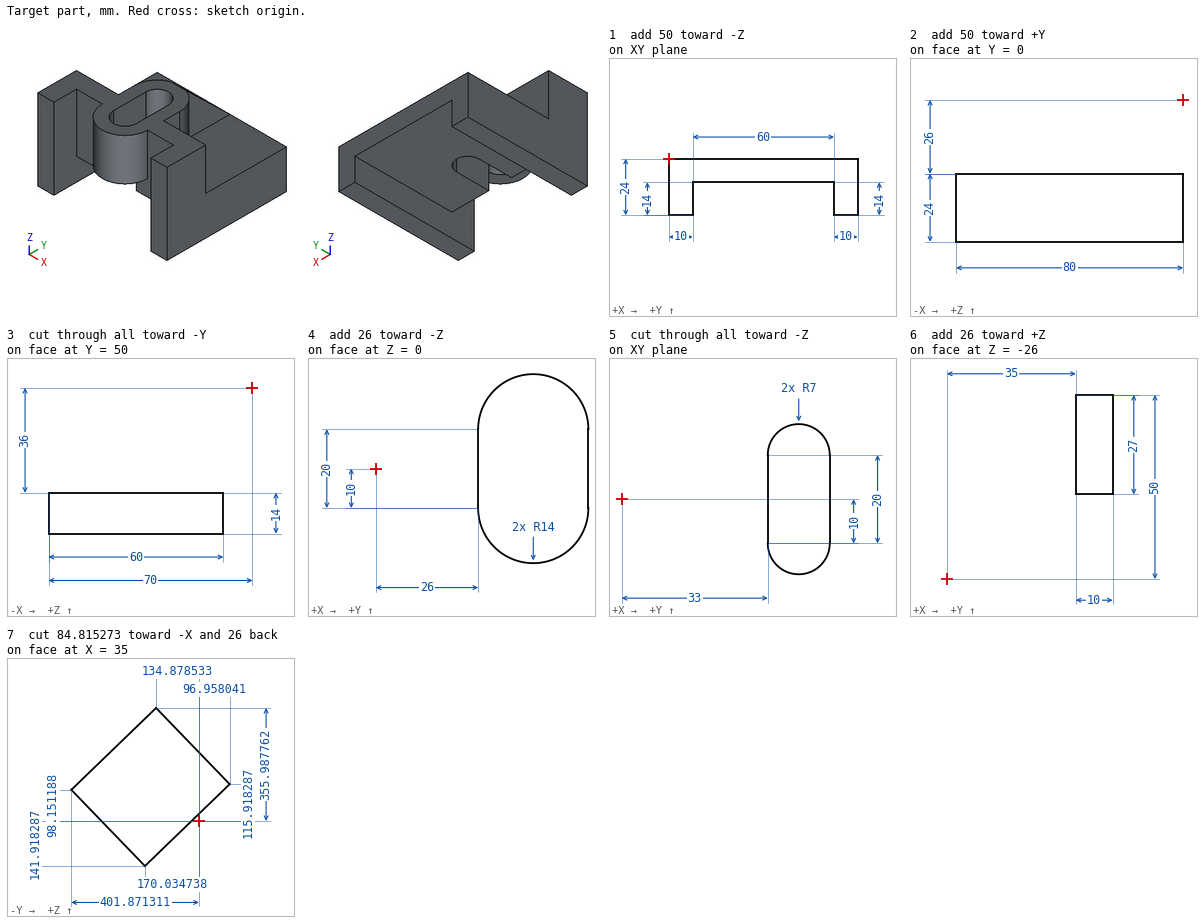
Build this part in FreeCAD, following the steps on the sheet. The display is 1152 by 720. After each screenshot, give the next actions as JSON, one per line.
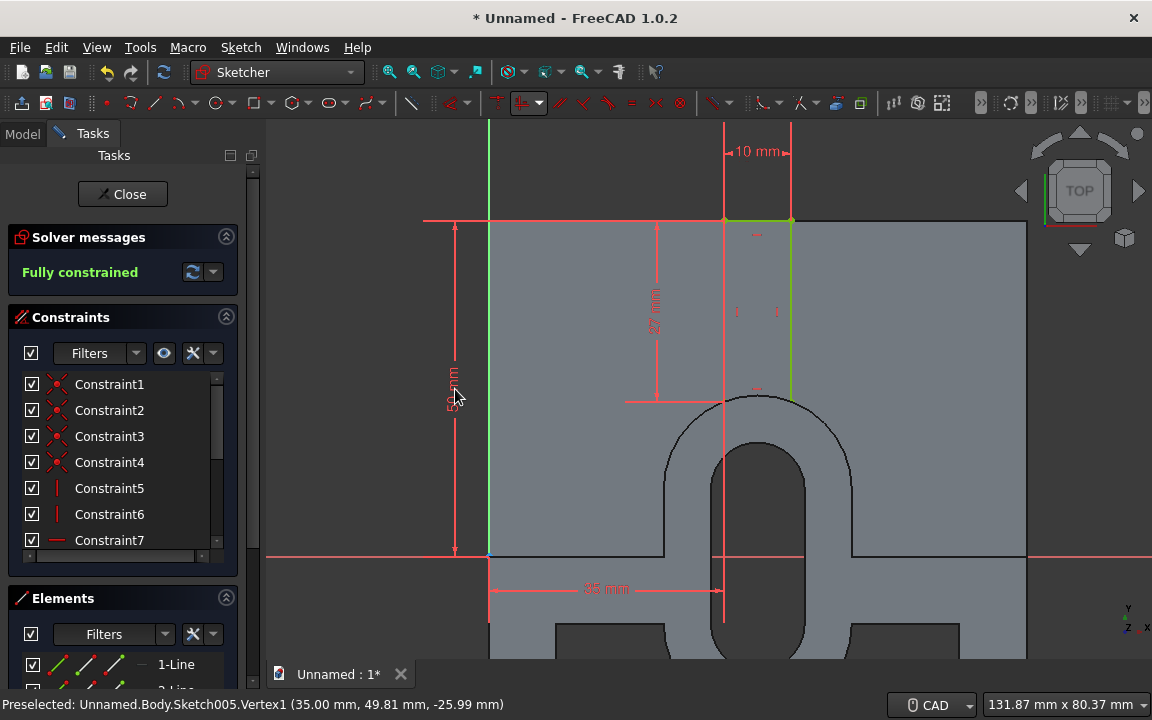
{"action": "left_click", "coordinate": [123, 194]}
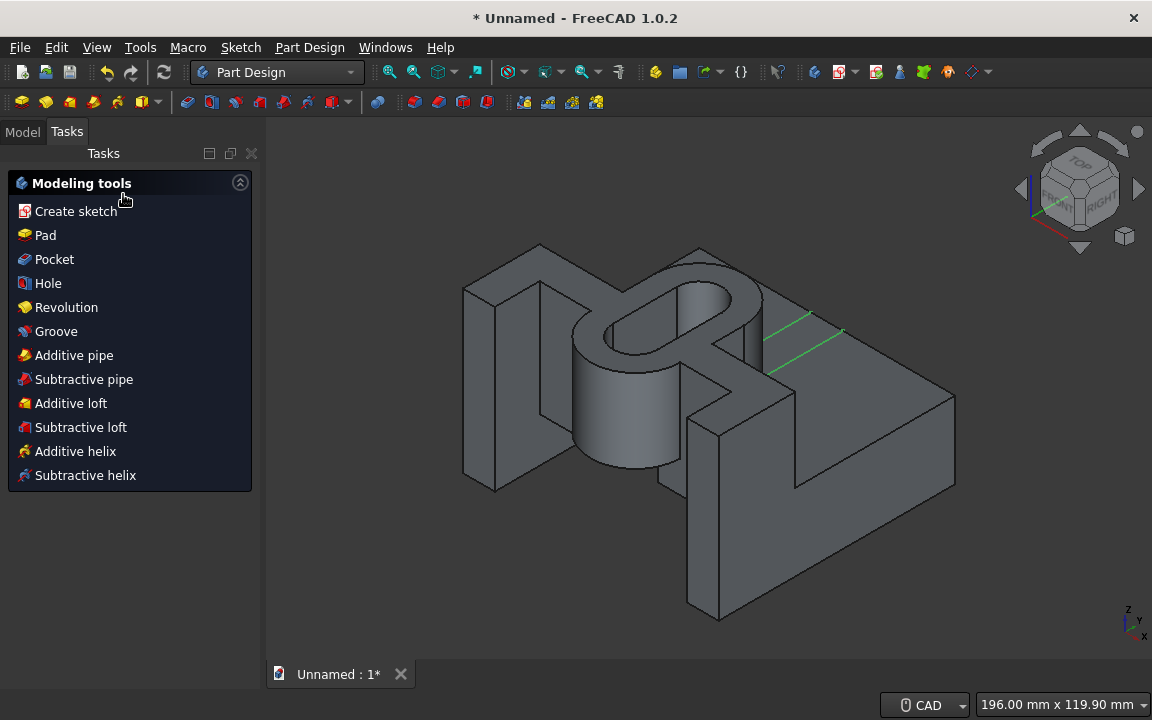
{"action": "left_click", "coordinate": [22, 102]}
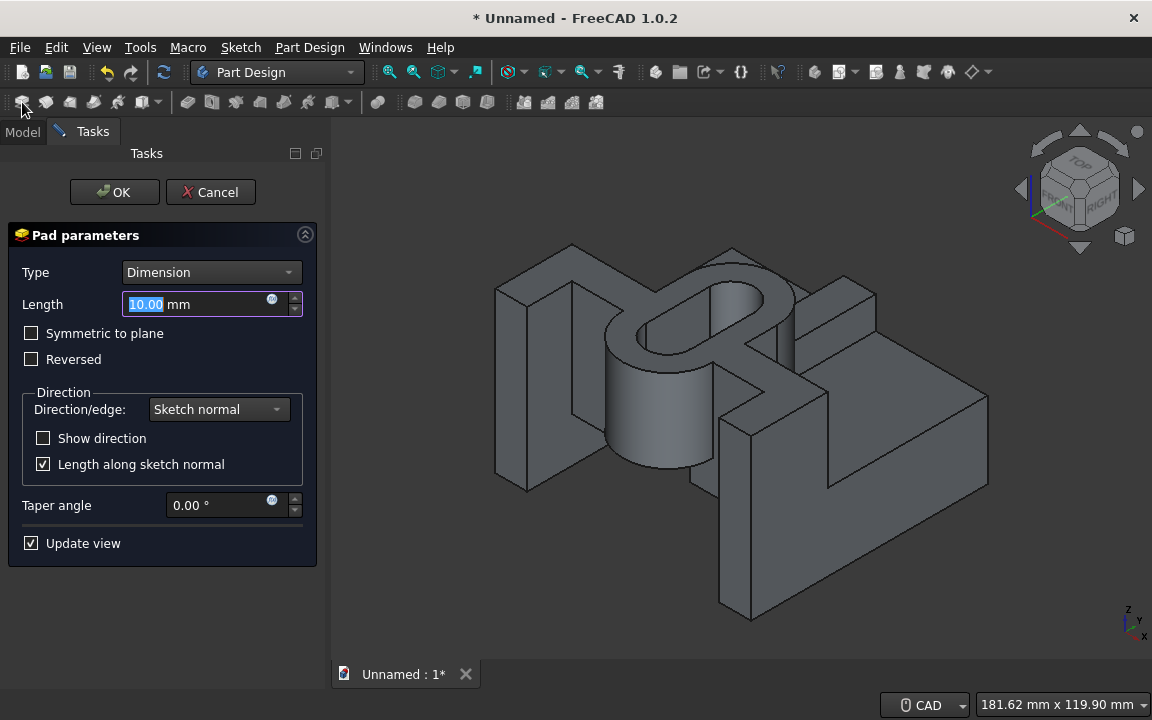
{"action": "type", "text": "26"}
{"action": "key", "text": "Tab"}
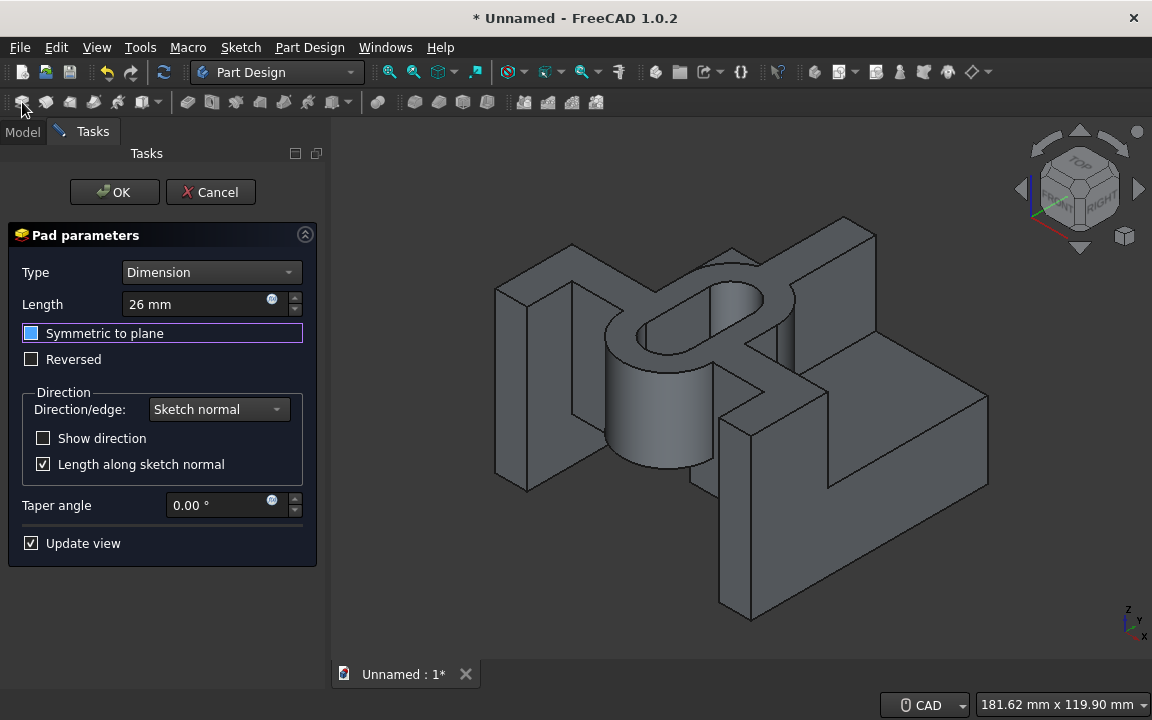
{"action": "left_click", "coordinate": [115, 192]}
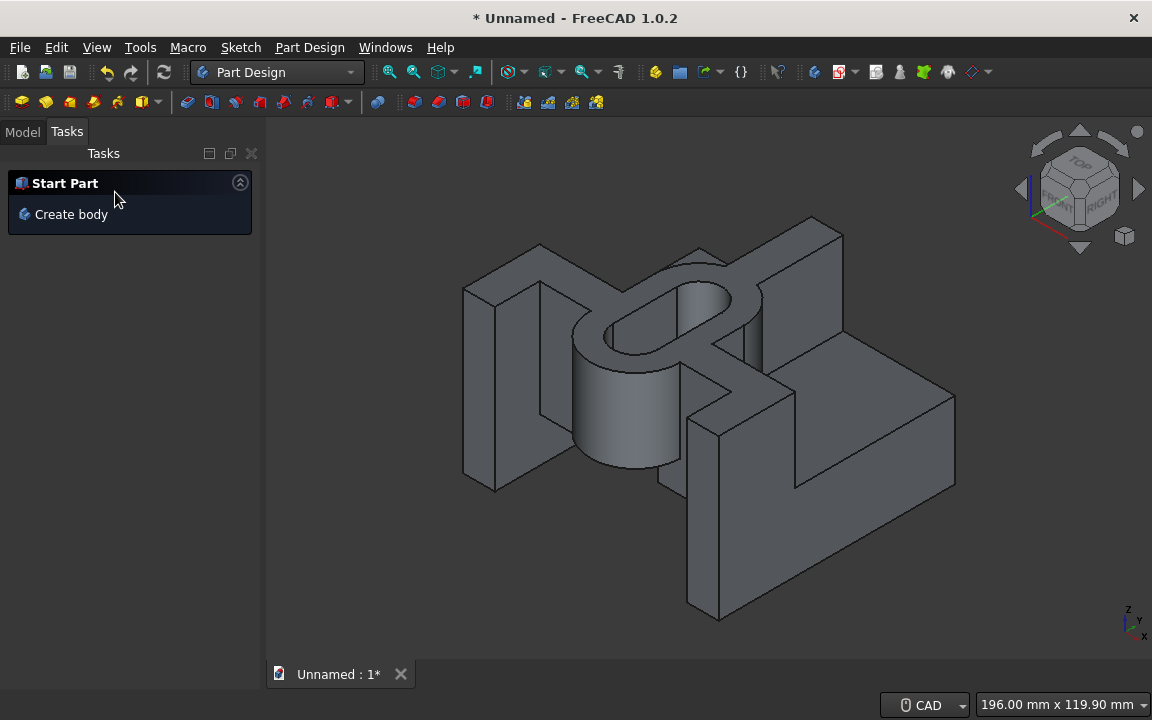
{"action": "key", "text": "6"}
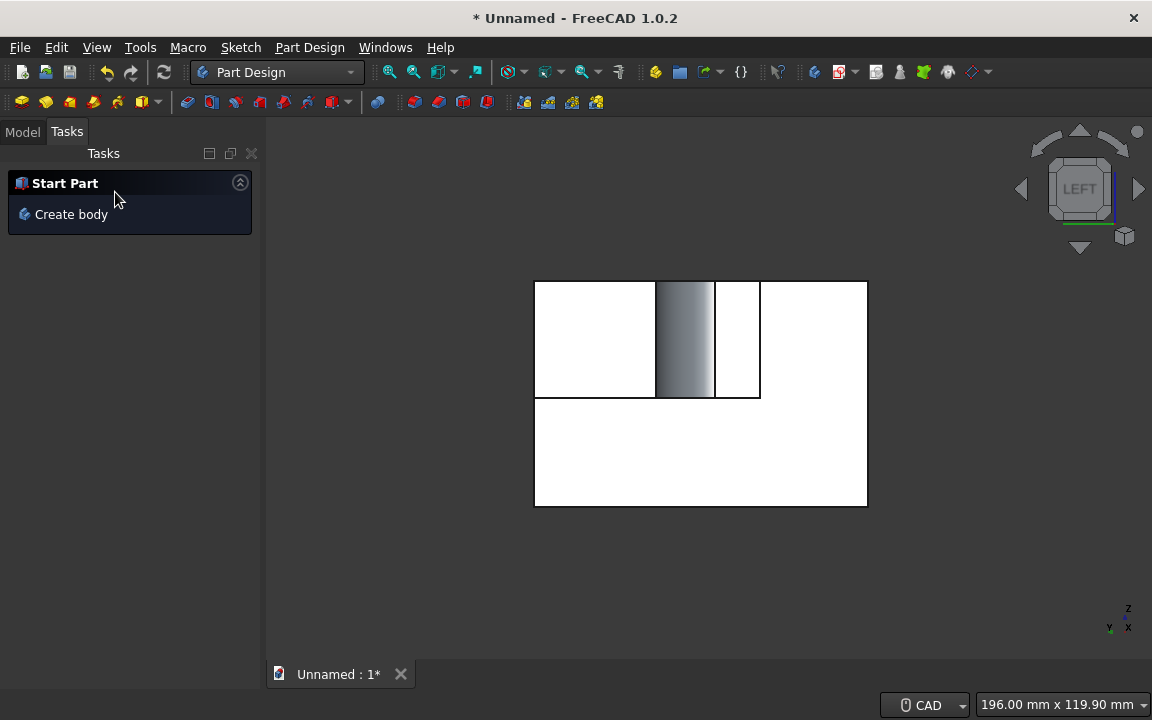
{"action": "key", "text": "v f"}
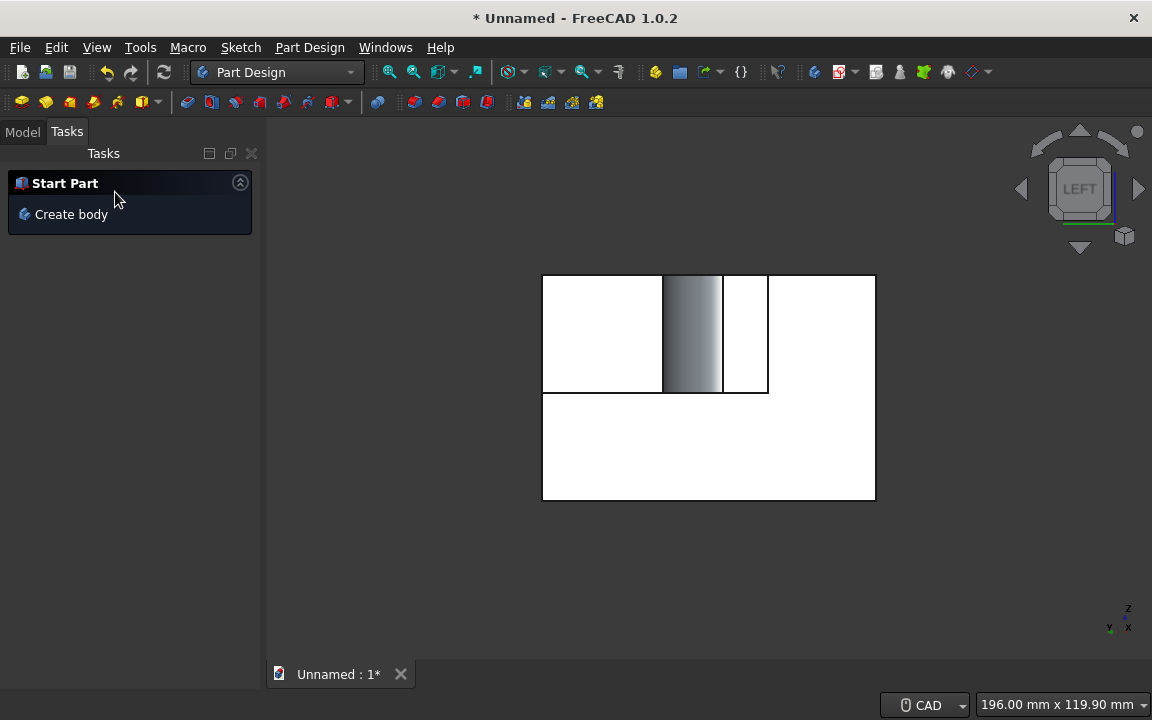
{"action": "left_click", "coordinate": [603, 333]}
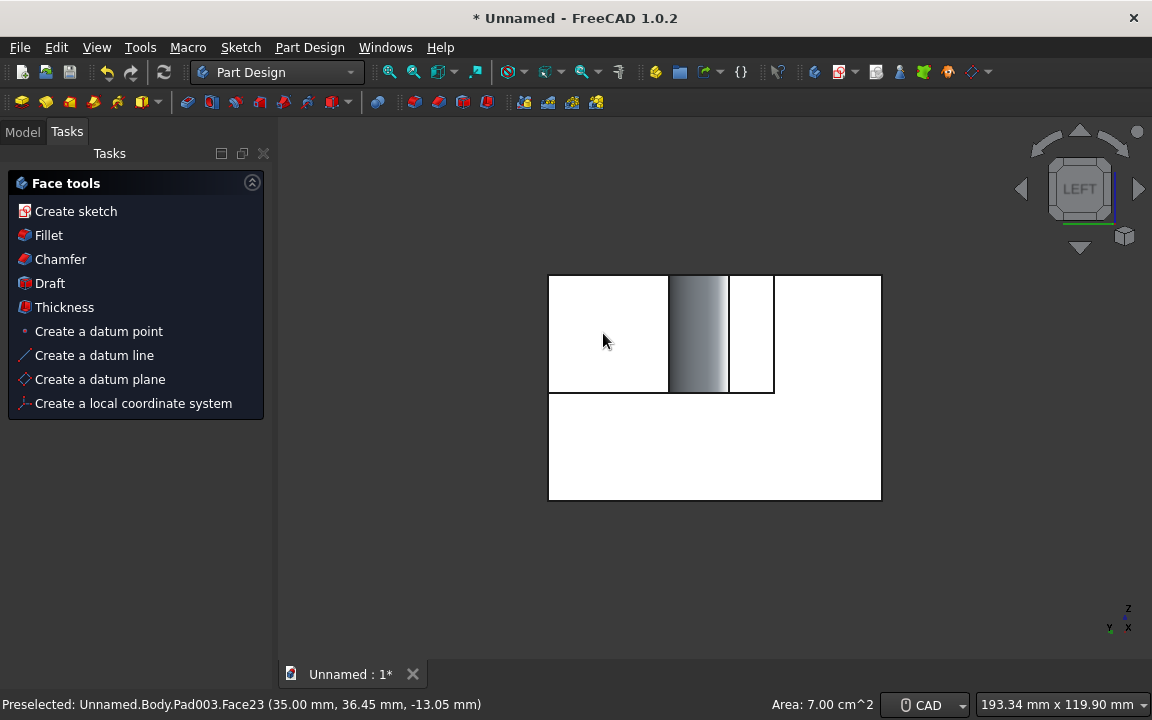
{"action": "left_click", "coordinate": [840, 72]}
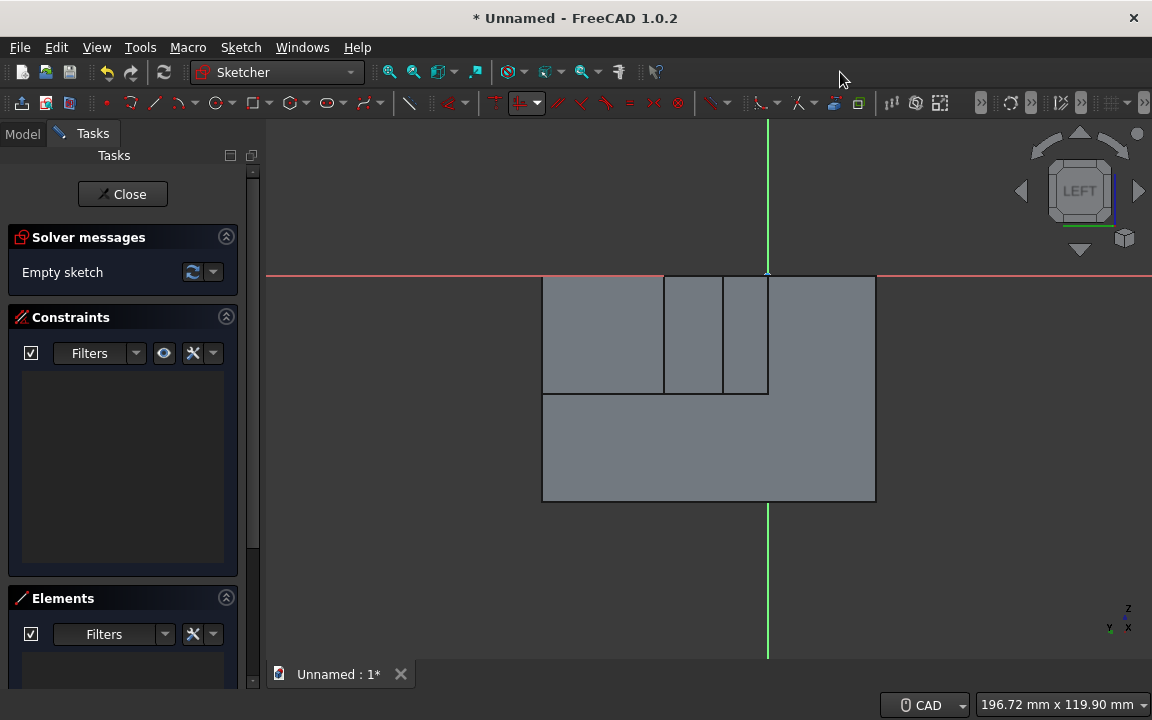
{"action": "scroll", "coordinate": [751, 507], "scroll_direction": "down", "scroll_amount": 9}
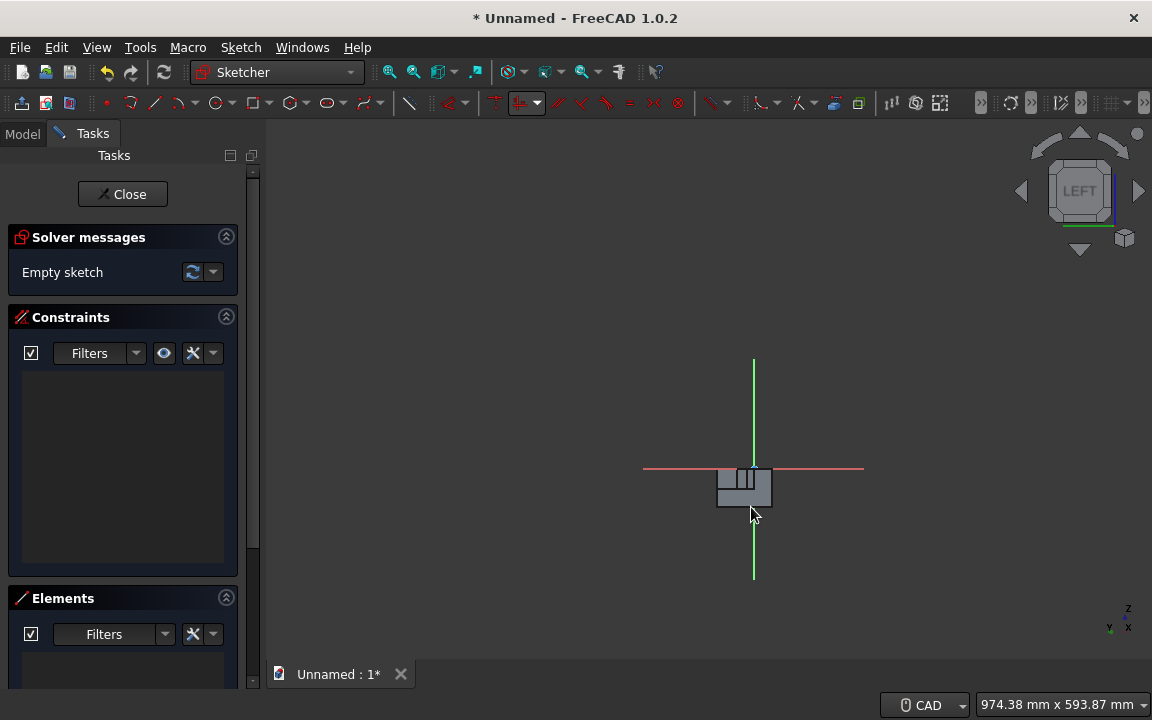
{"action": "left_click", "coordinate": [132, 104]}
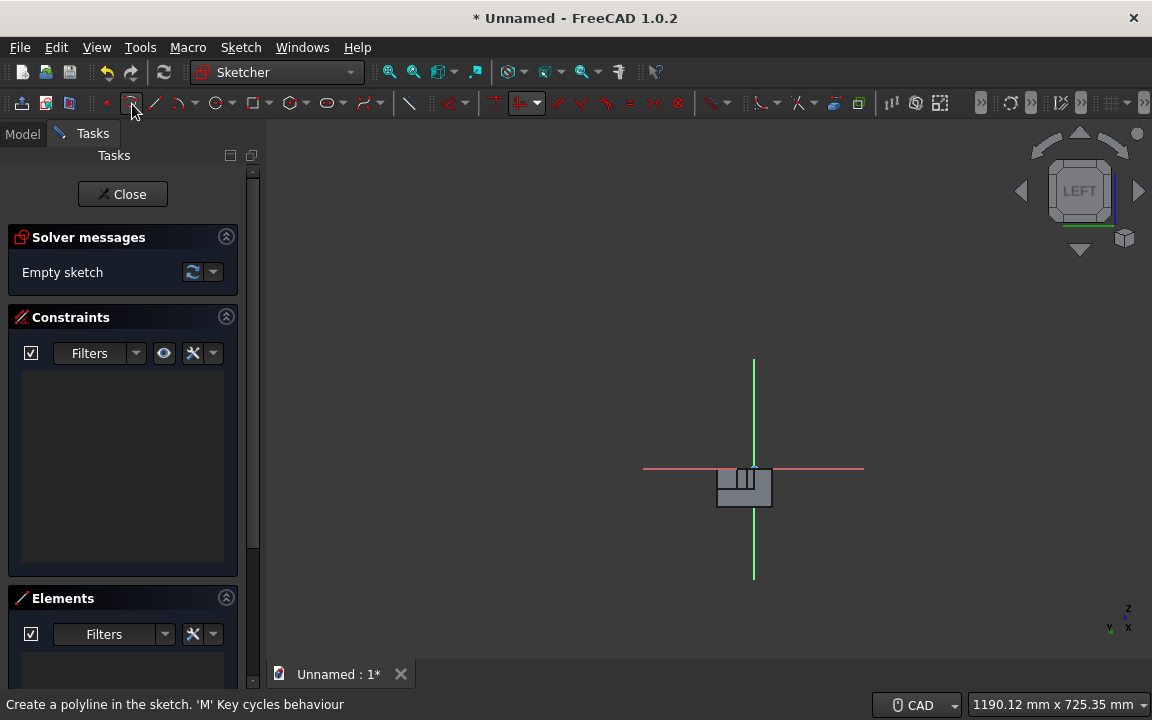
{"action": "left_click", "coordinate": [826, 383]}
{"action": "left_click", "coordinate": [654, 204]}
{"action": "left_click", "coordinate": [455, 396]}
{"action": "left_click", "coordinate": [628, 575]}
{"action": "left_click", "coordinate": [826, 384]}
{"action": "key", "text": "Escape"}
{"action": "key", "text": "Escape"}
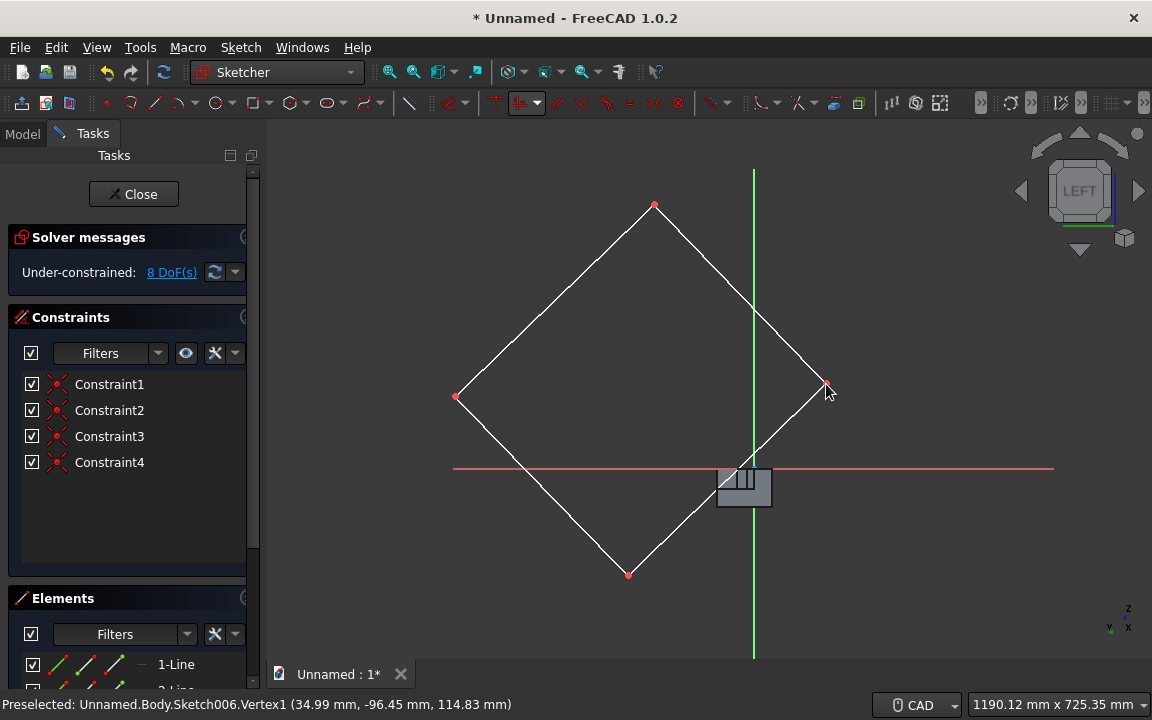
{"action": "key", "text": "d"}